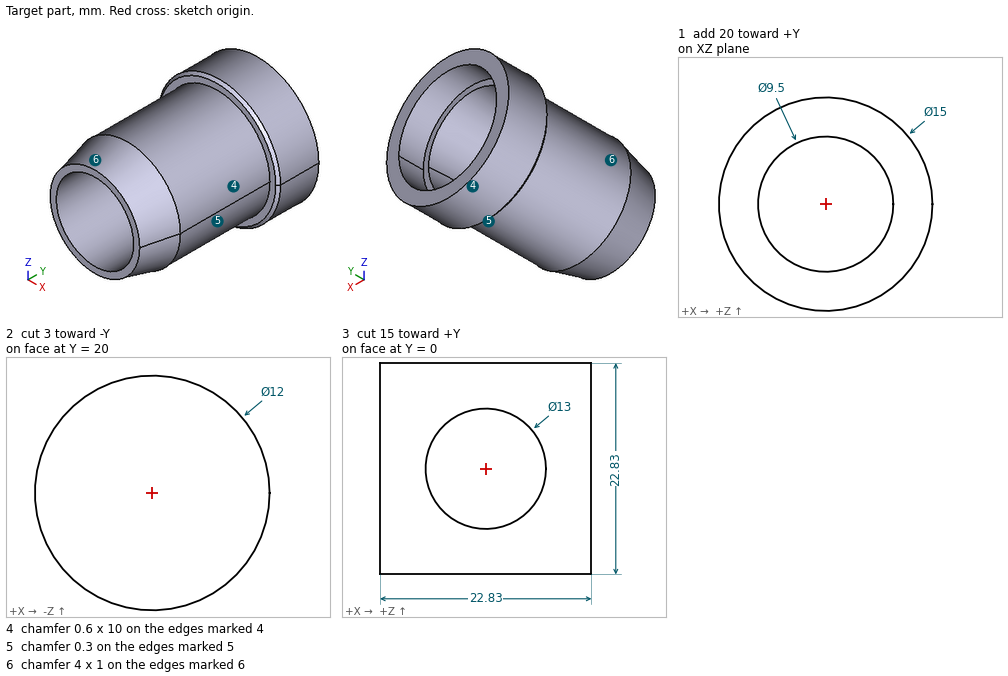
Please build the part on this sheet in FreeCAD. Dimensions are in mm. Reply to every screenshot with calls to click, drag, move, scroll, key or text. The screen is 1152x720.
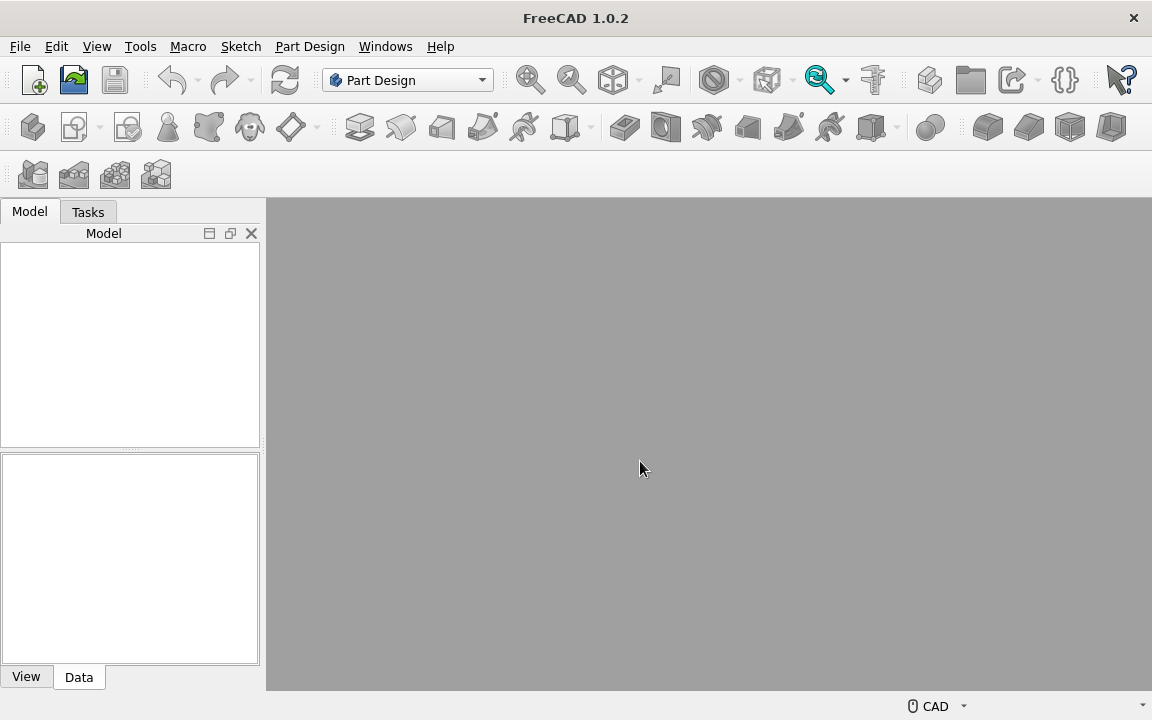
click(33, 80)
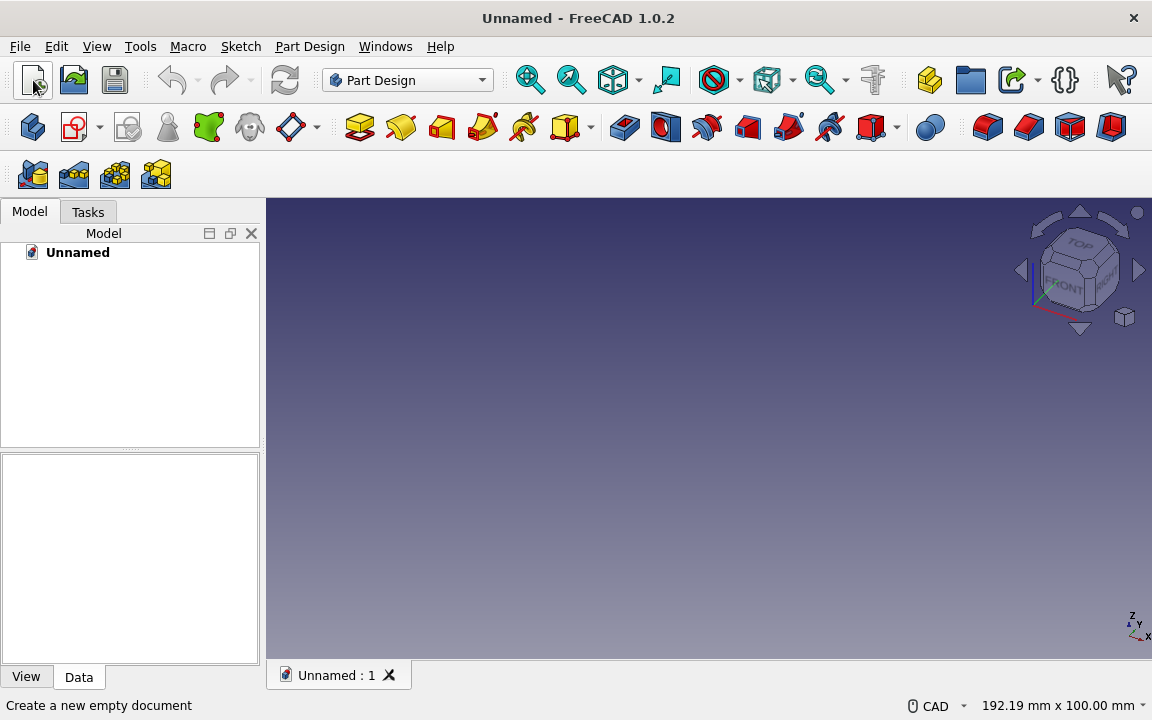
click(74, 128)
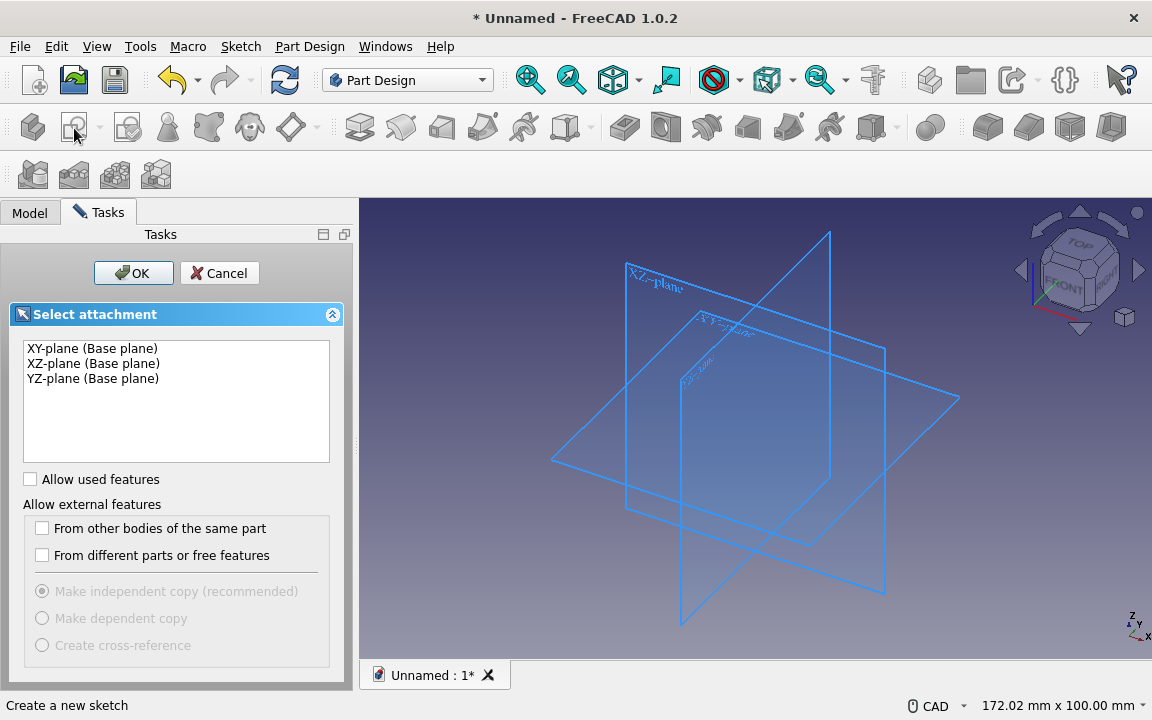
click(84, 364)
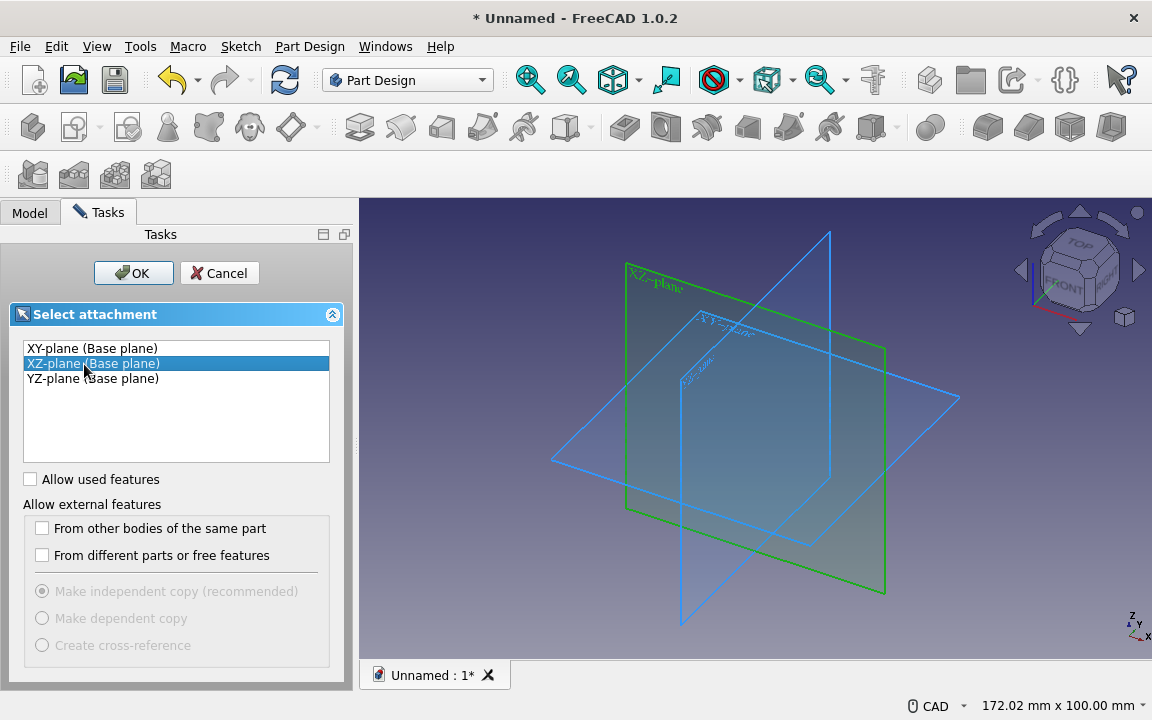
click(134, 273)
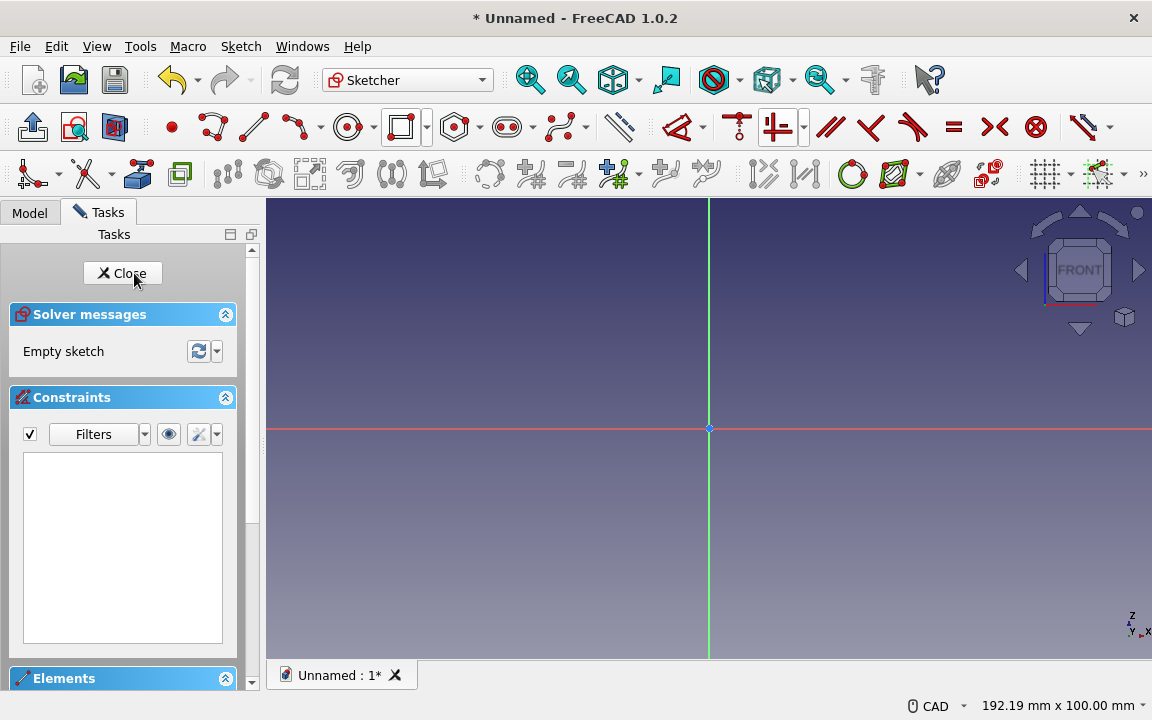
scroll(731, 429, up, 7)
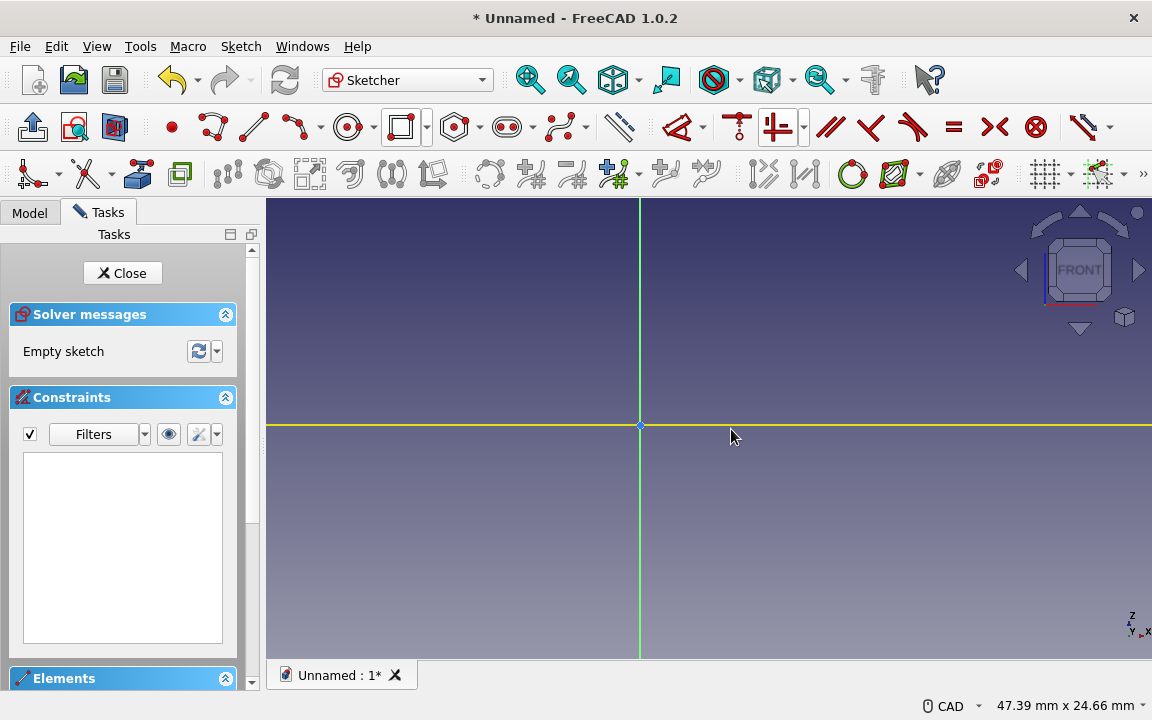
click(348, 128)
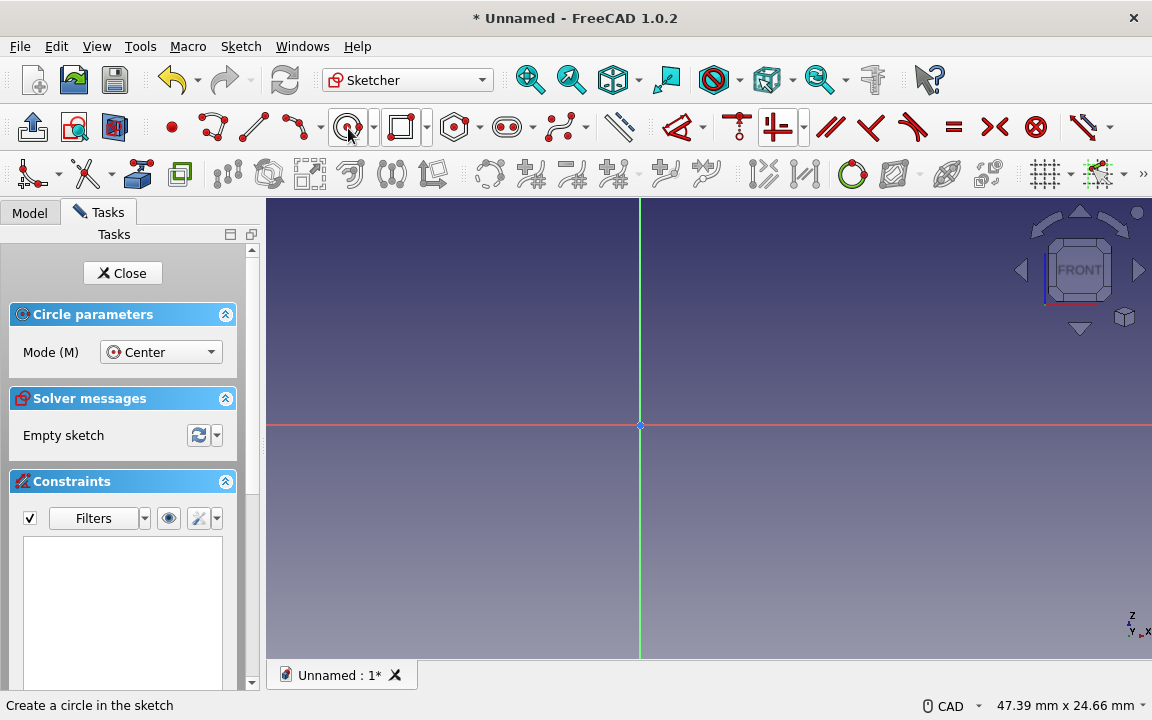
click(640, 425)
move(739, 326)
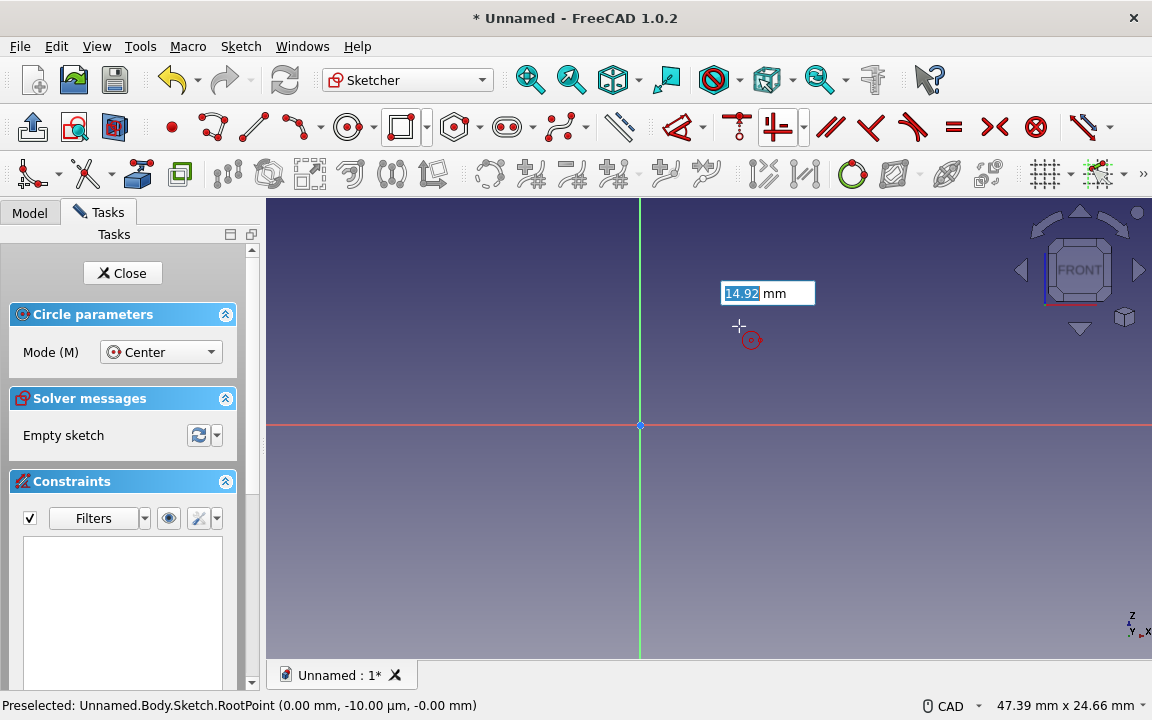
text(15)
key(Return)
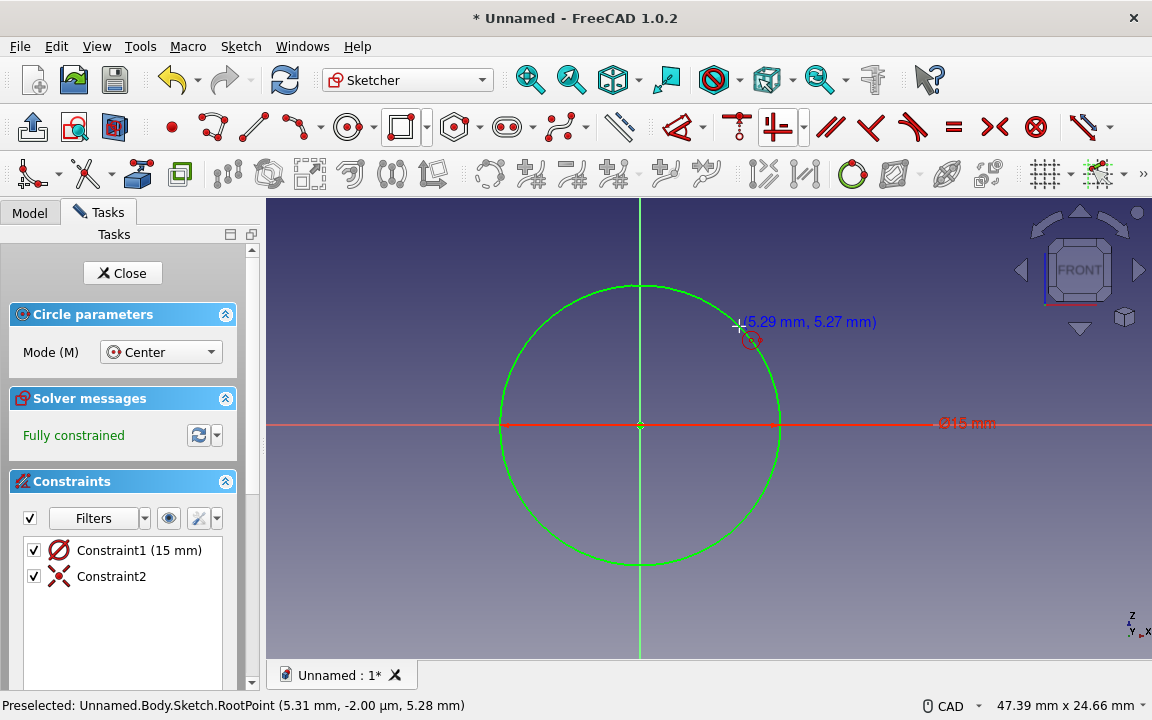
click(640, 425)
move(703, 363)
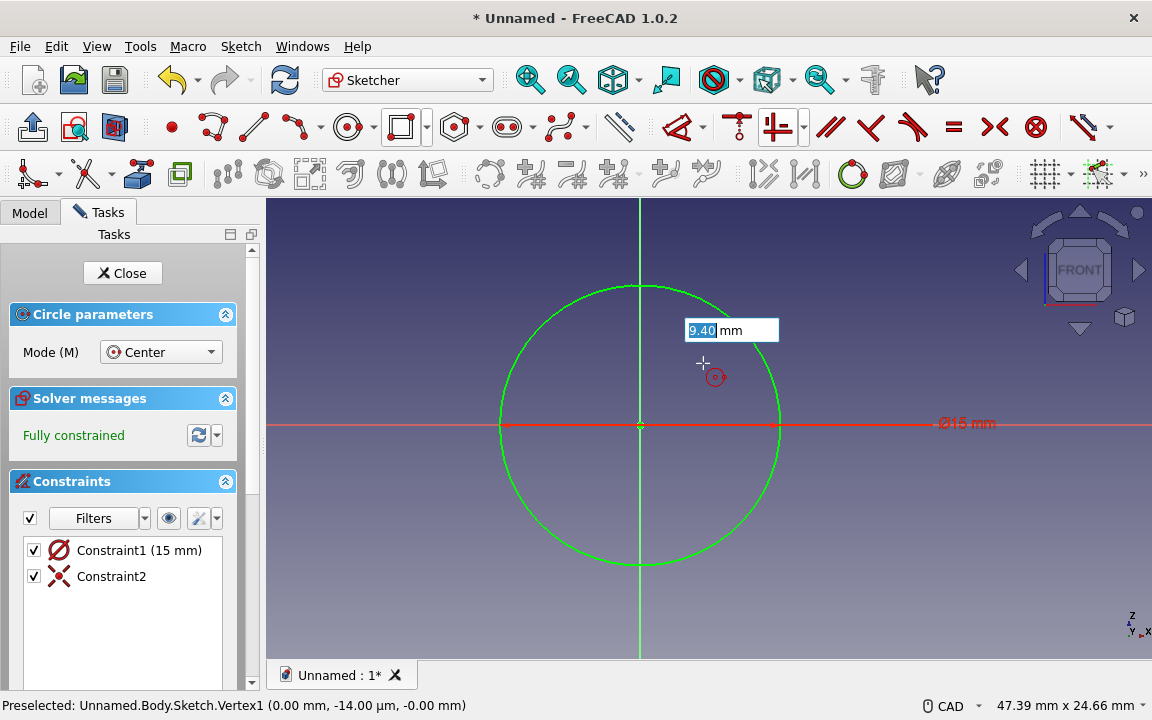
text(9.5)
key(Return)
key(Escape)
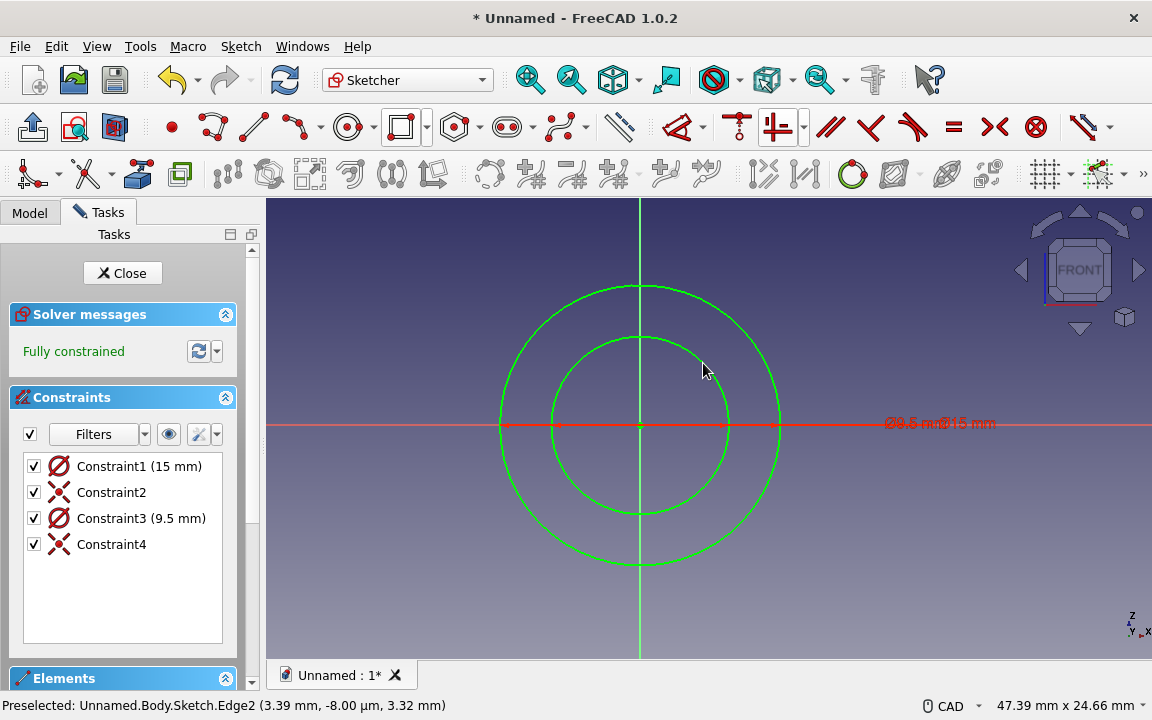
click(123, 273)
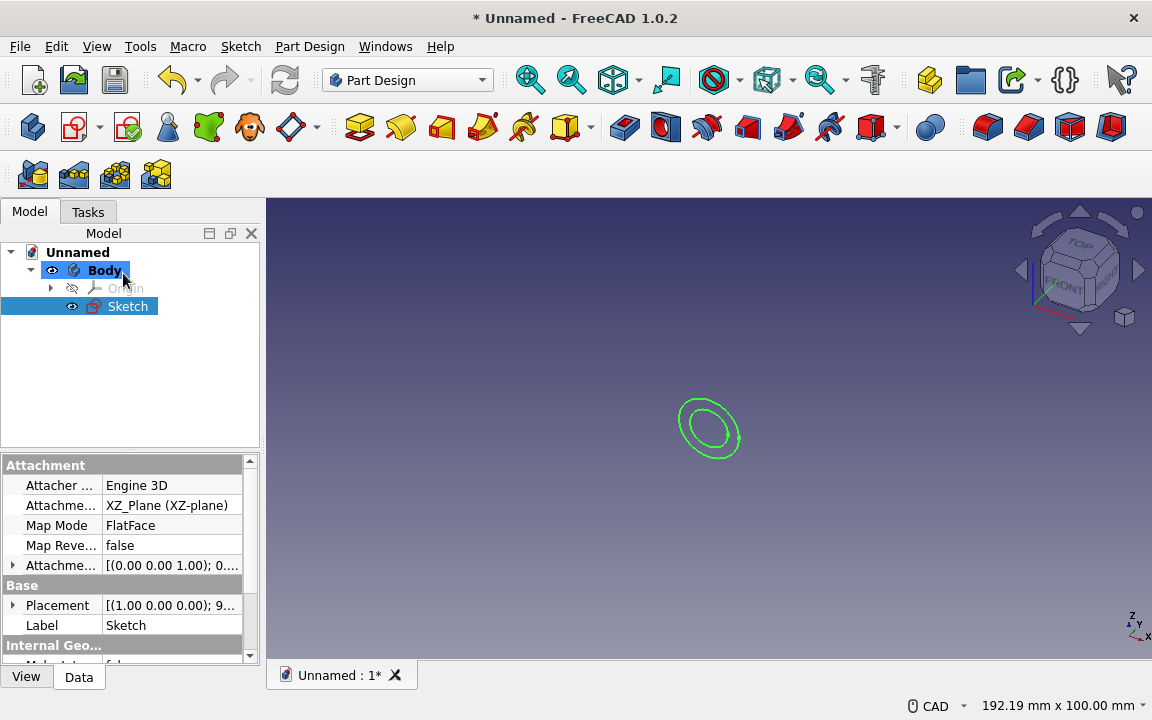
click(360, 128)